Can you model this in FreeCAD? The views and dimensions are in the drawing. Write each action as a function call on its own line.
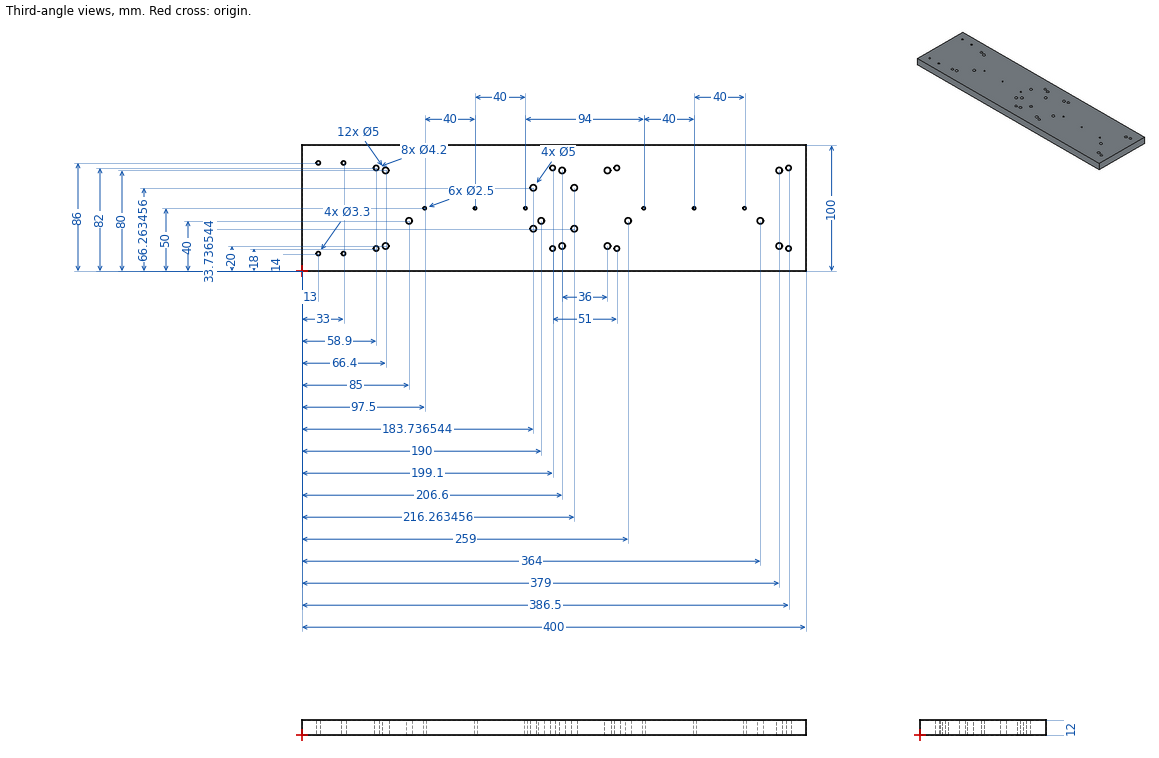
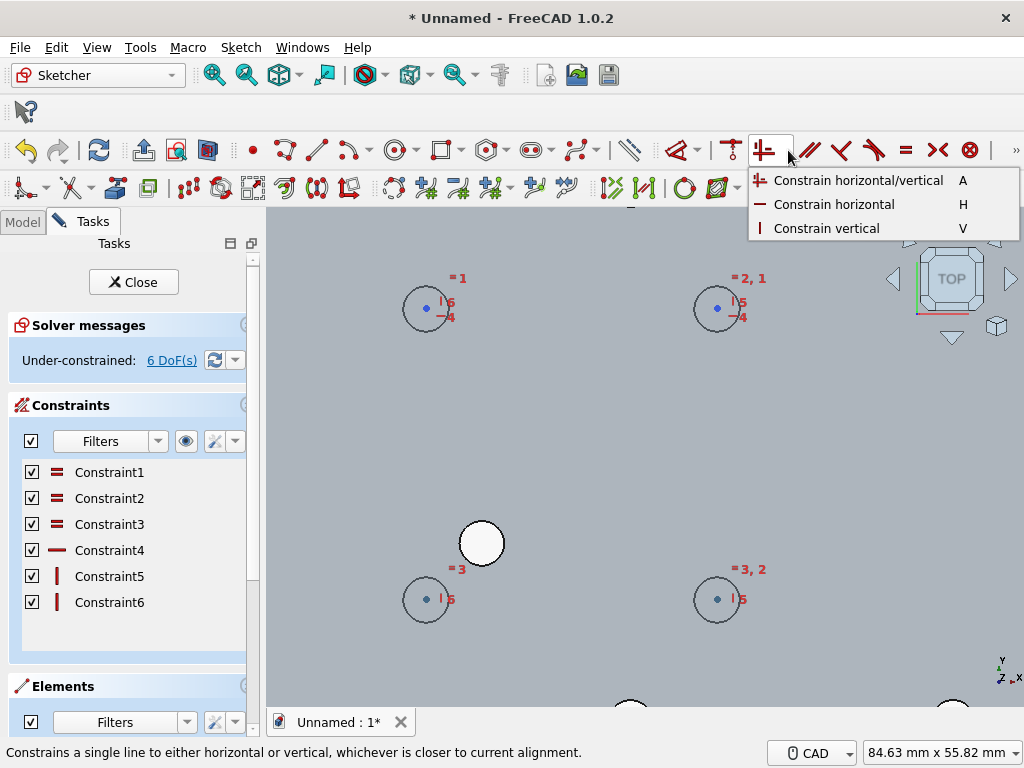
click(884, 204)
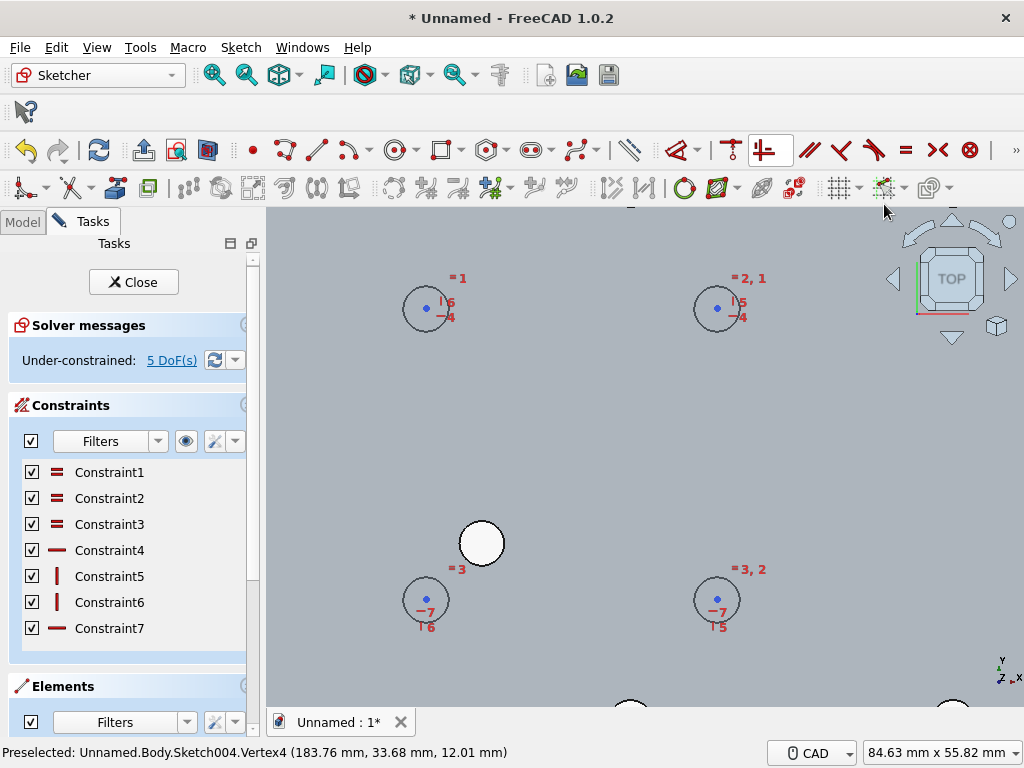
click(676, 150)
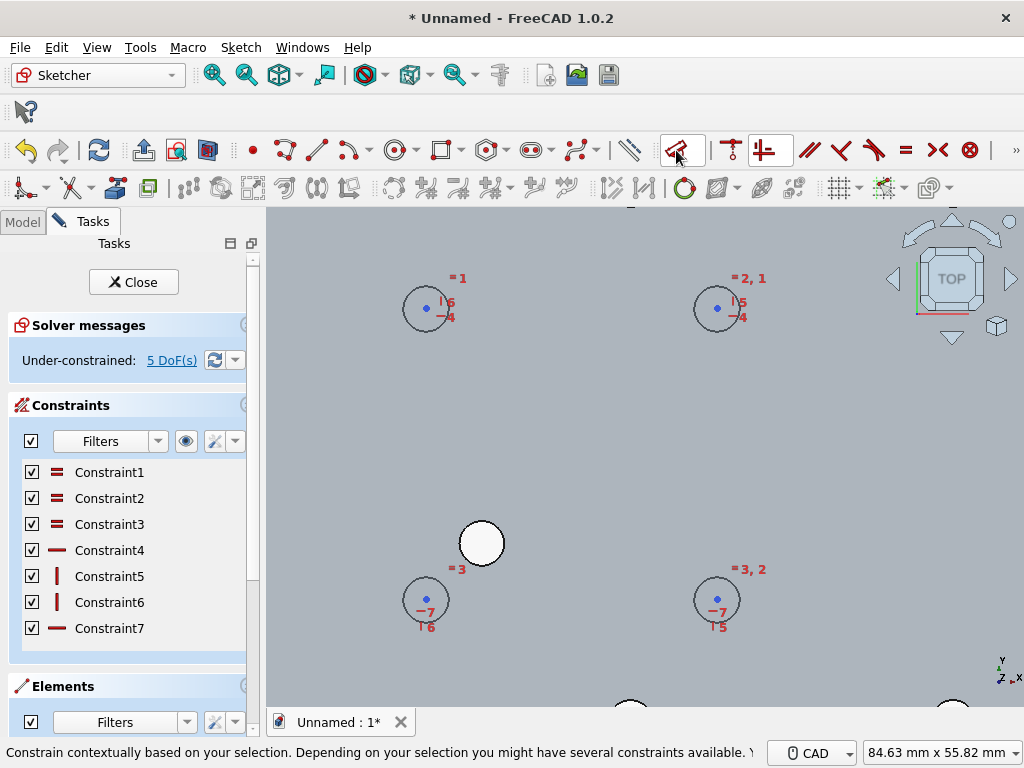
click(442, 293)
click(465, 270)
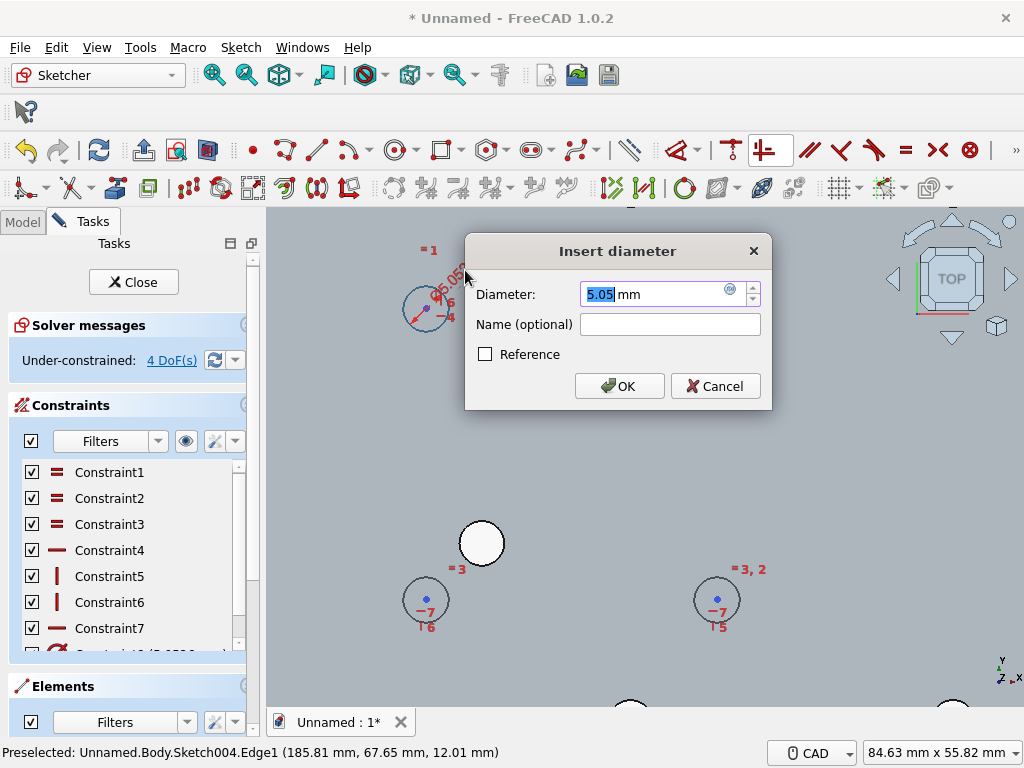
text(5)
key(Return)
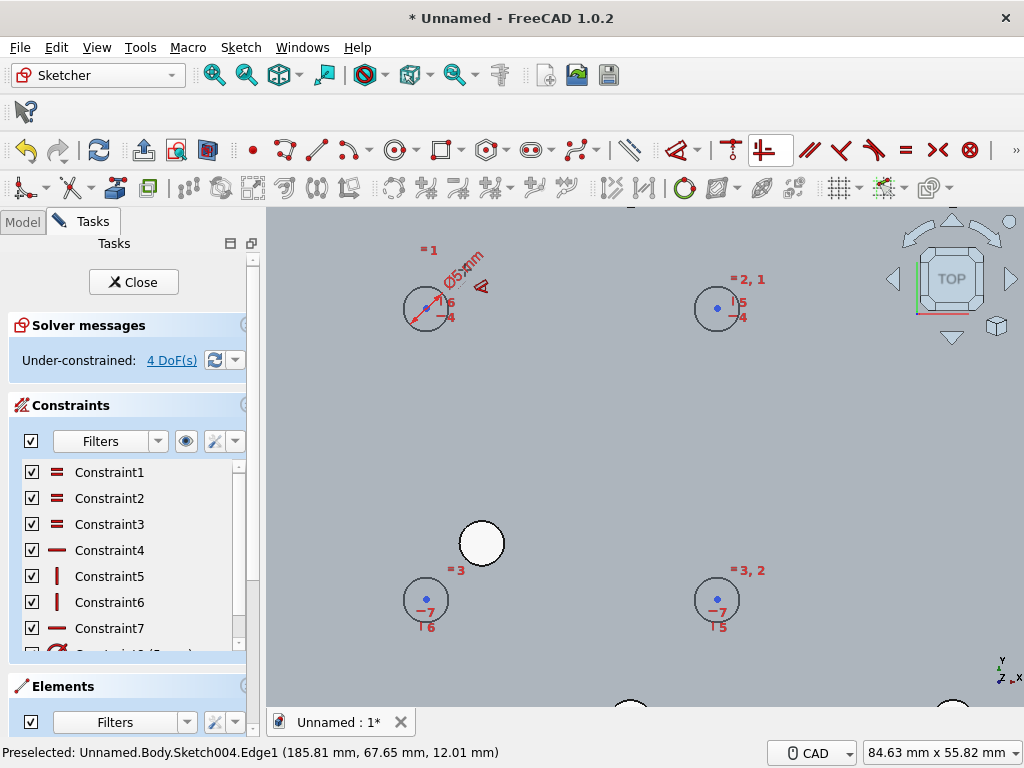
click(426, 309)
click(460, 494)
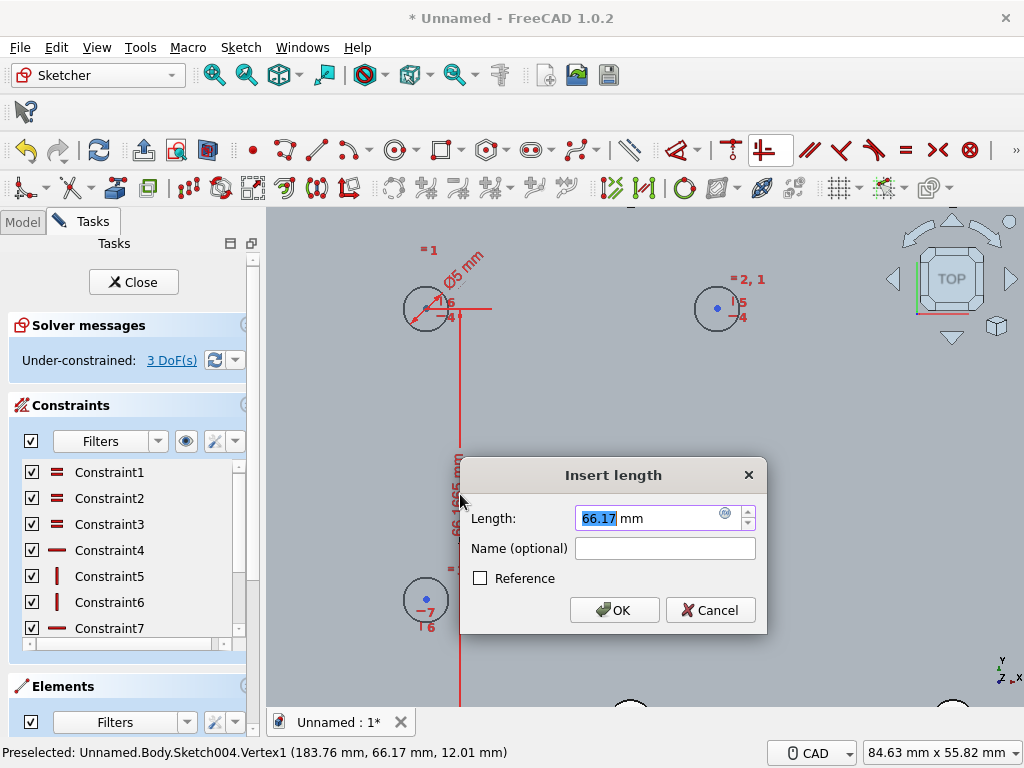
text(66.263456)
key(Return)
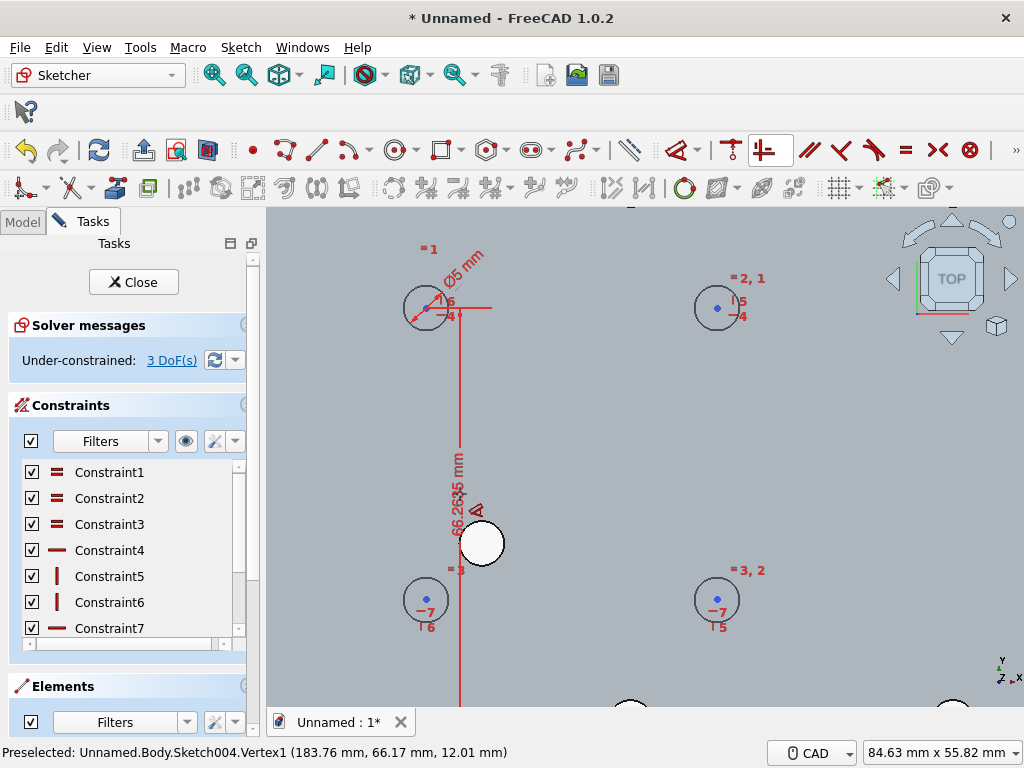
click(717, 600)
click(751, 639)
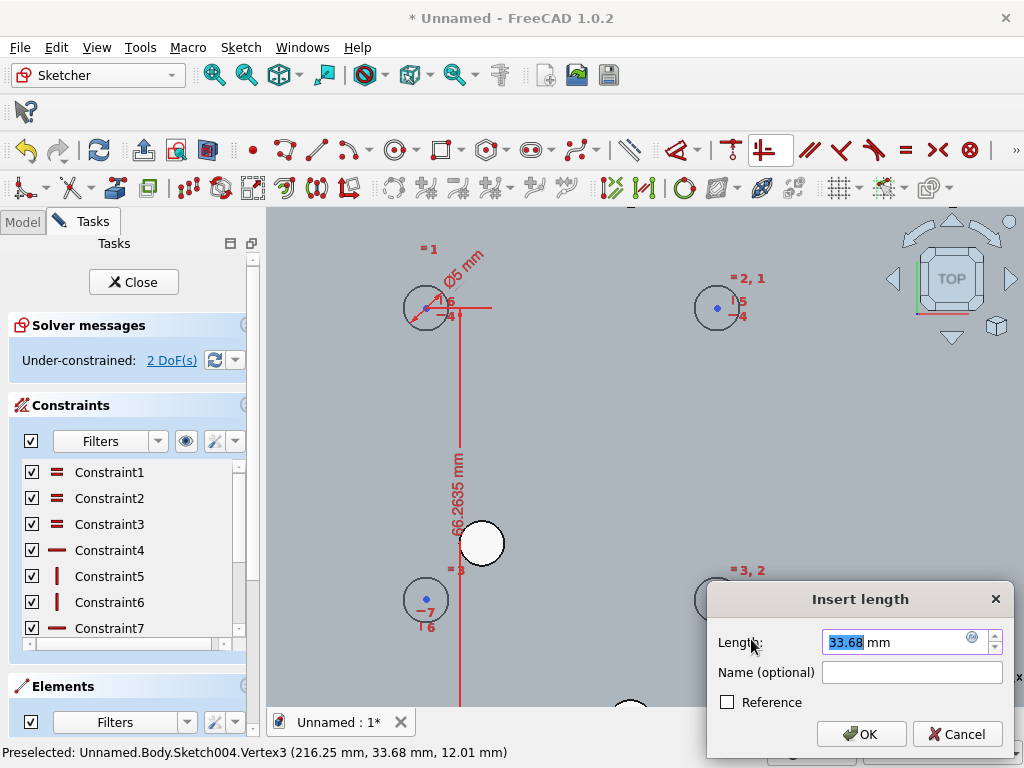
text(33.736544)
key(Return)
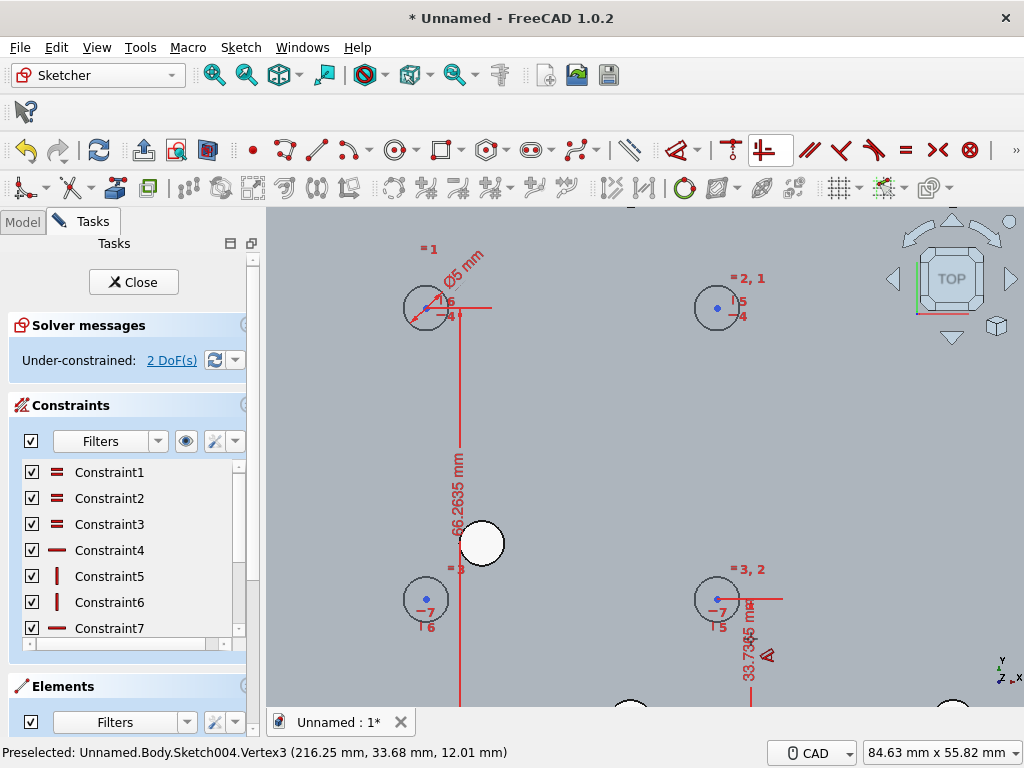
click(426, 308)
click(360, 274)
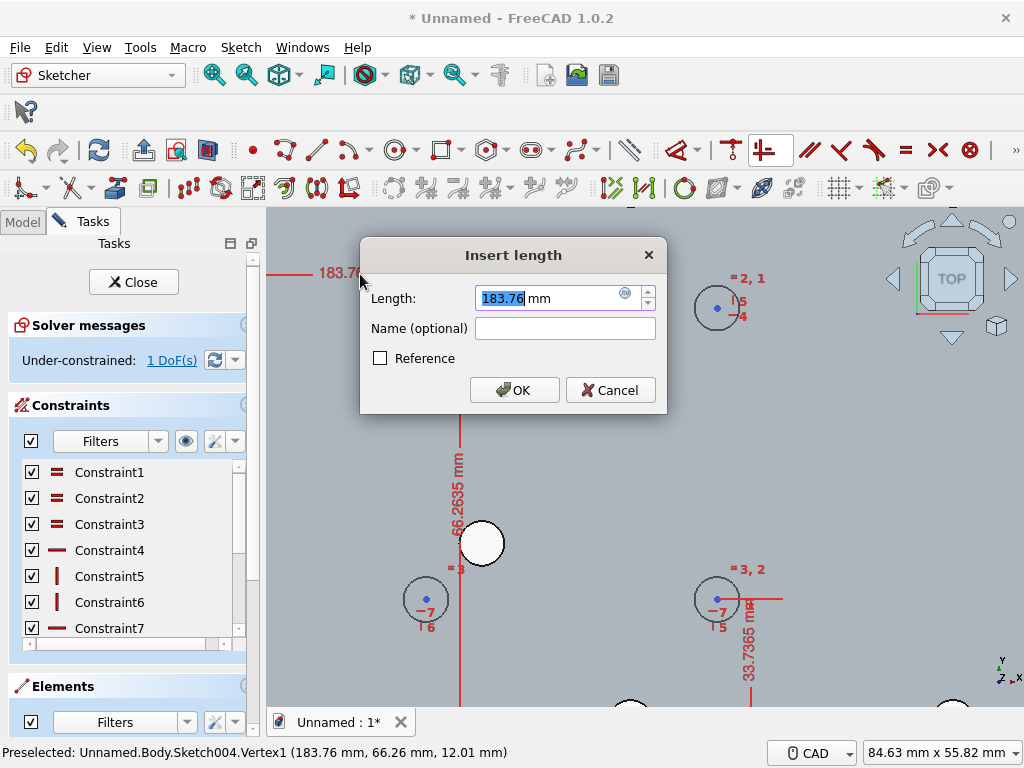
text(183.736544)
key(Return)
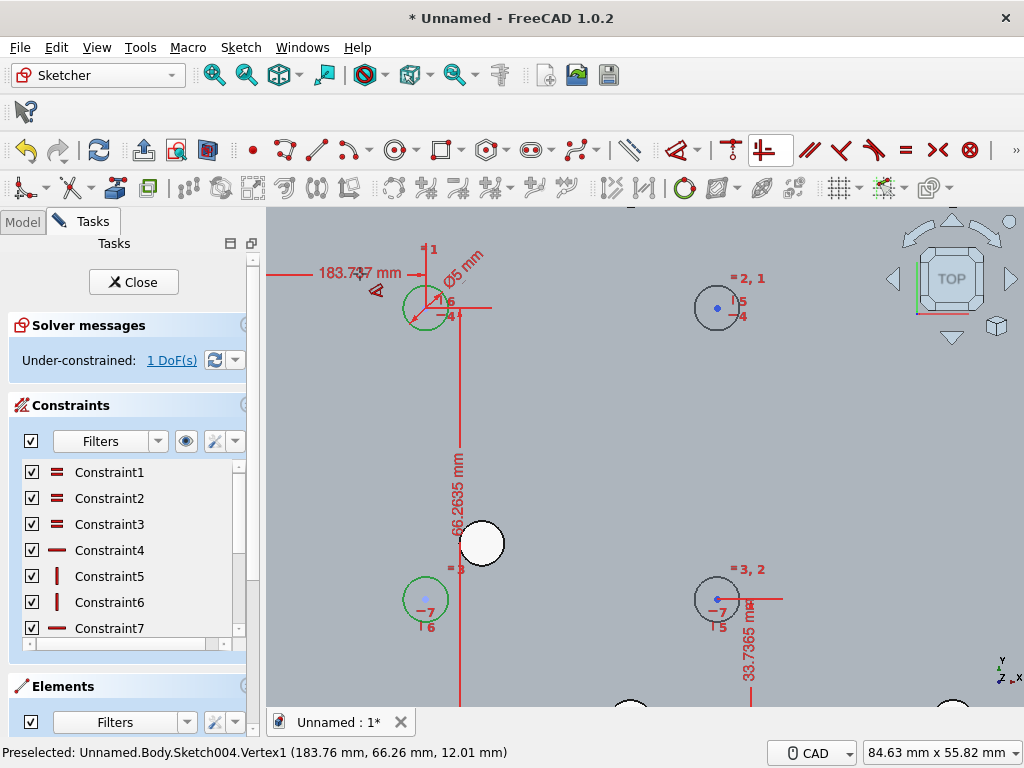
click(717, 308)
click(603, 274)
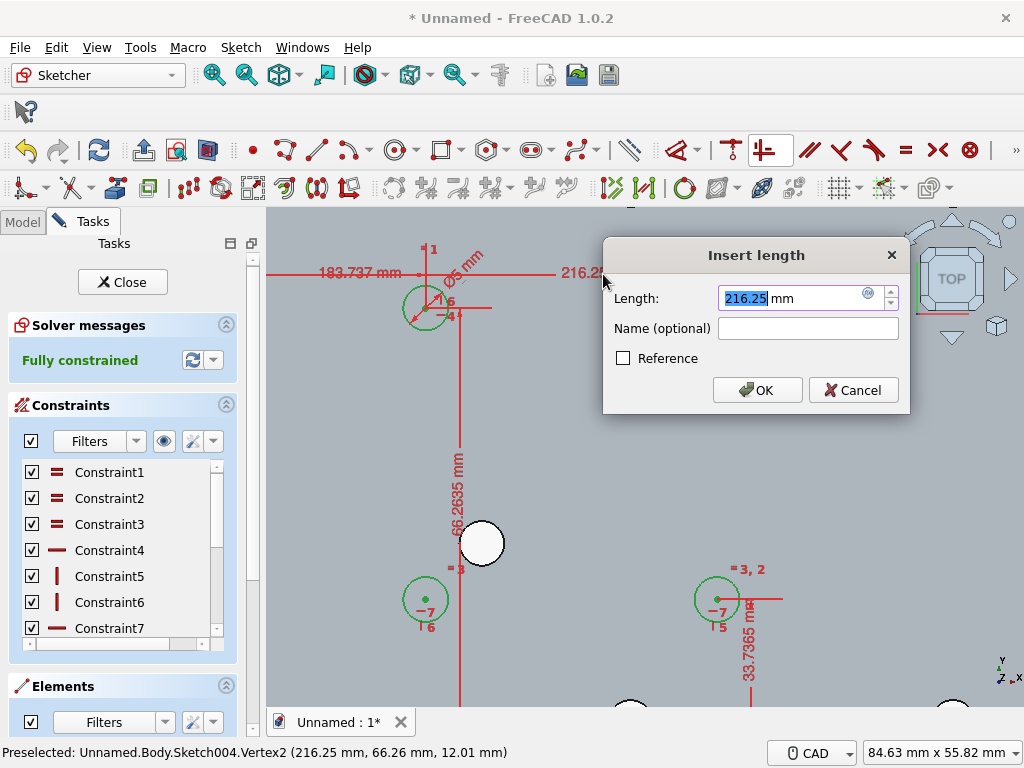
text(216.263456)
key(Return)
key(Escape)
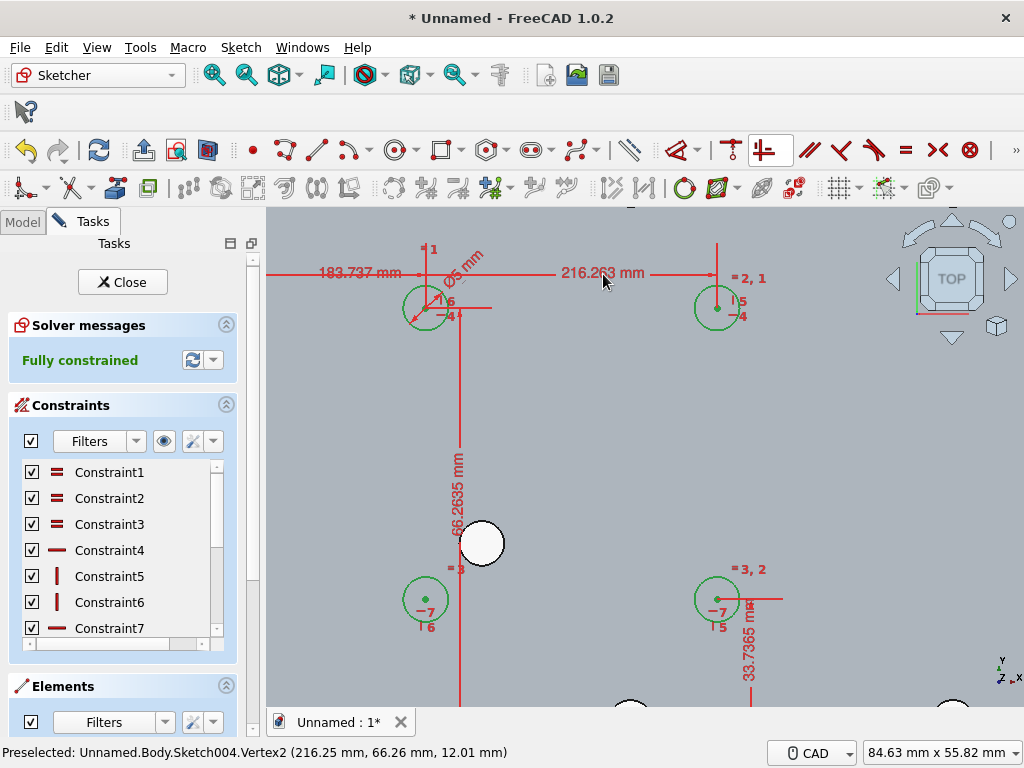
click(123, 282)